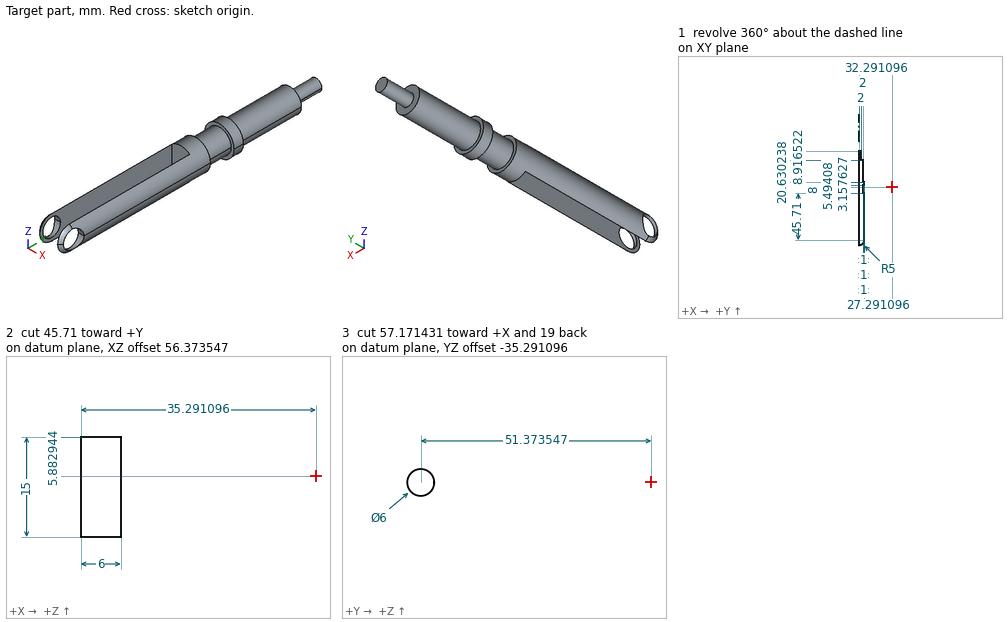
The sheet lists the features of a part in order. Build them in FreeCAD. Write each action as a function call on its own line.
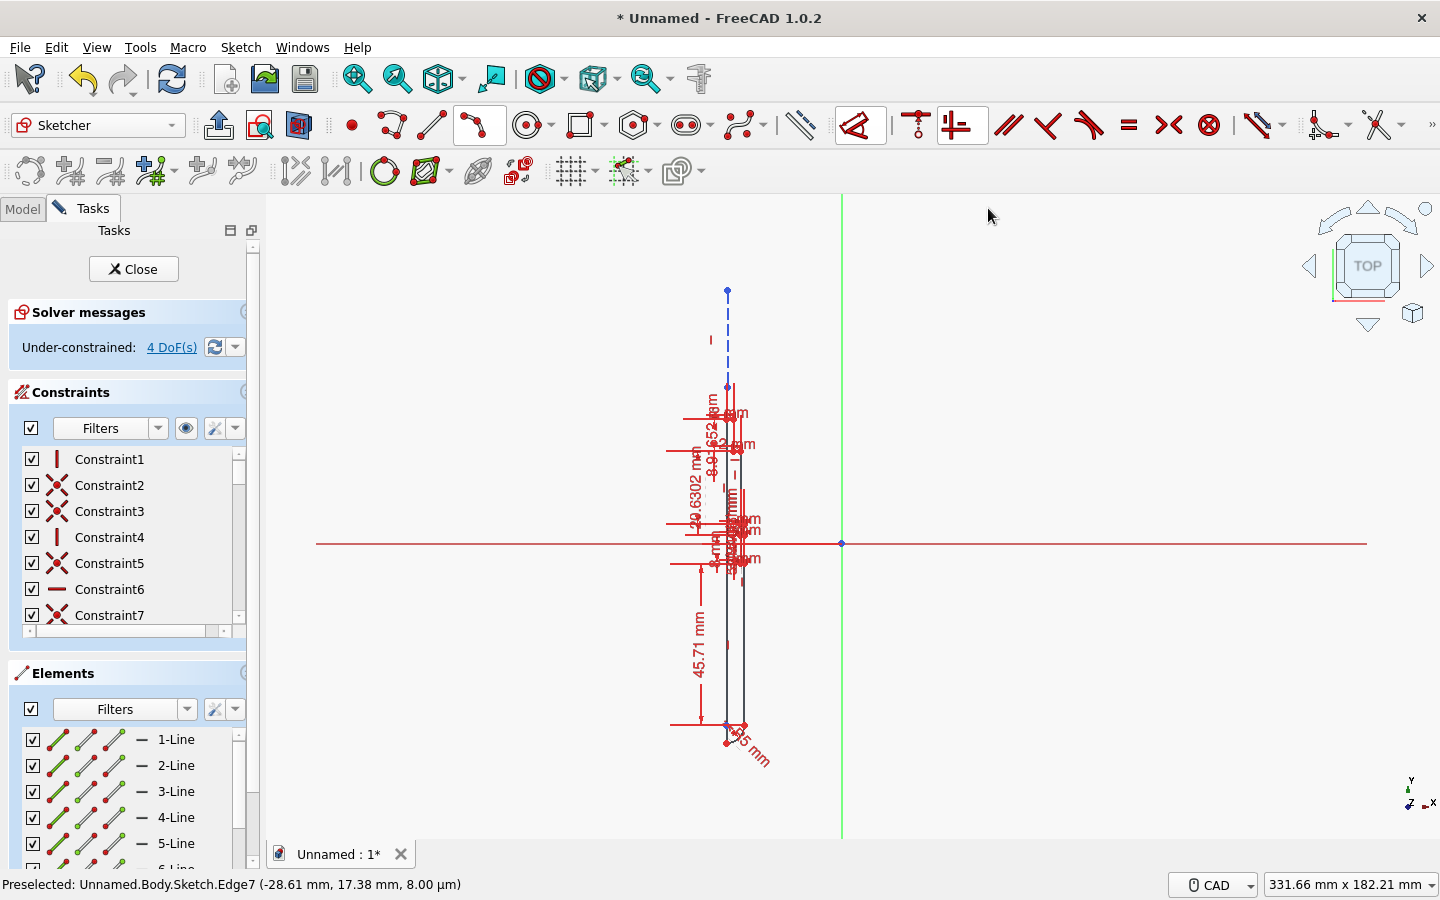
click(744, 725)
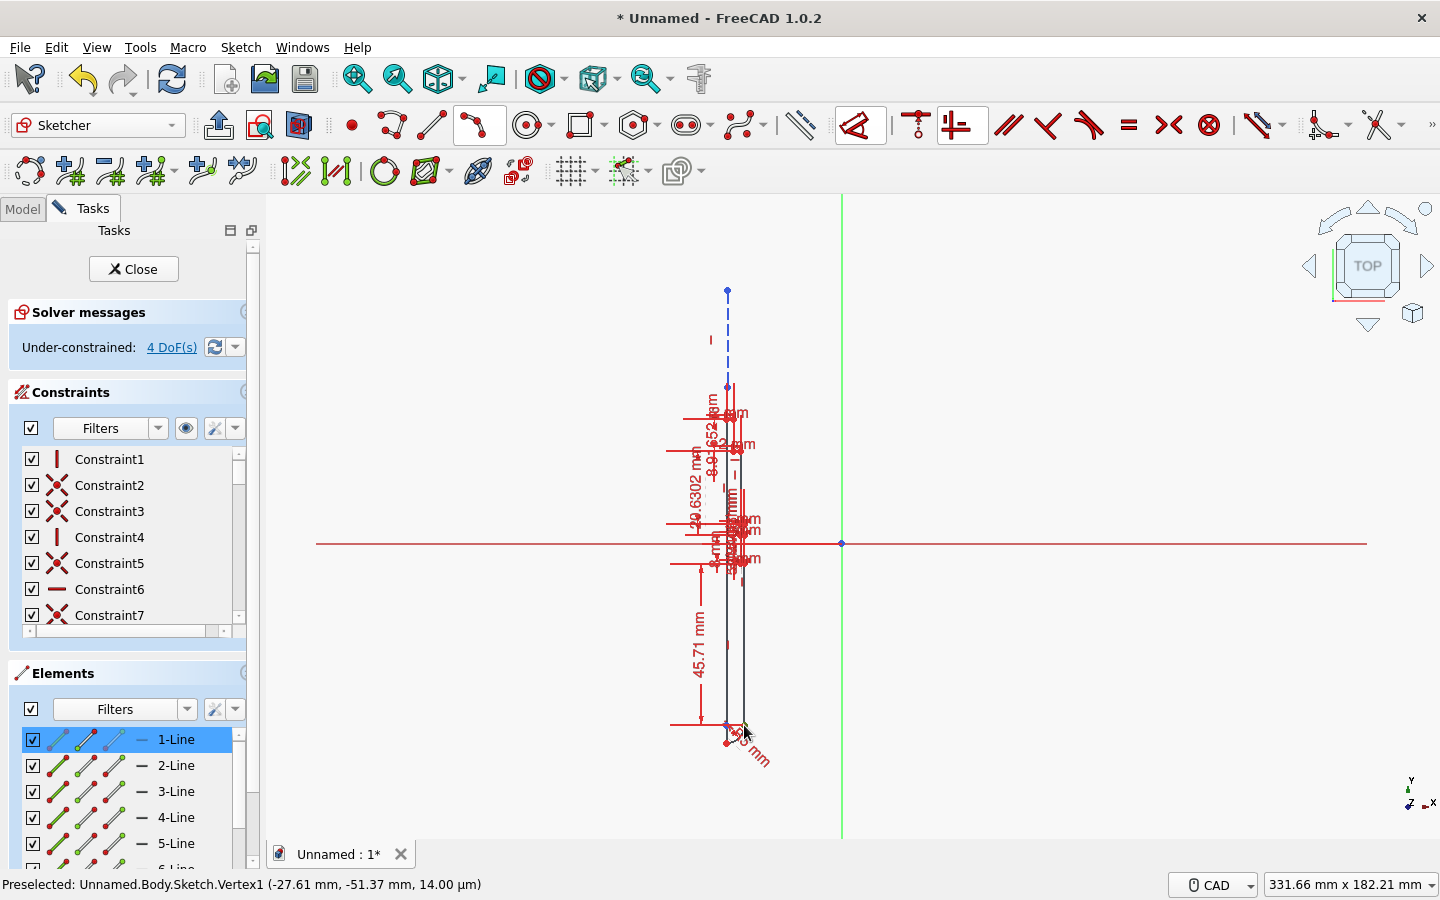
click(880, 126)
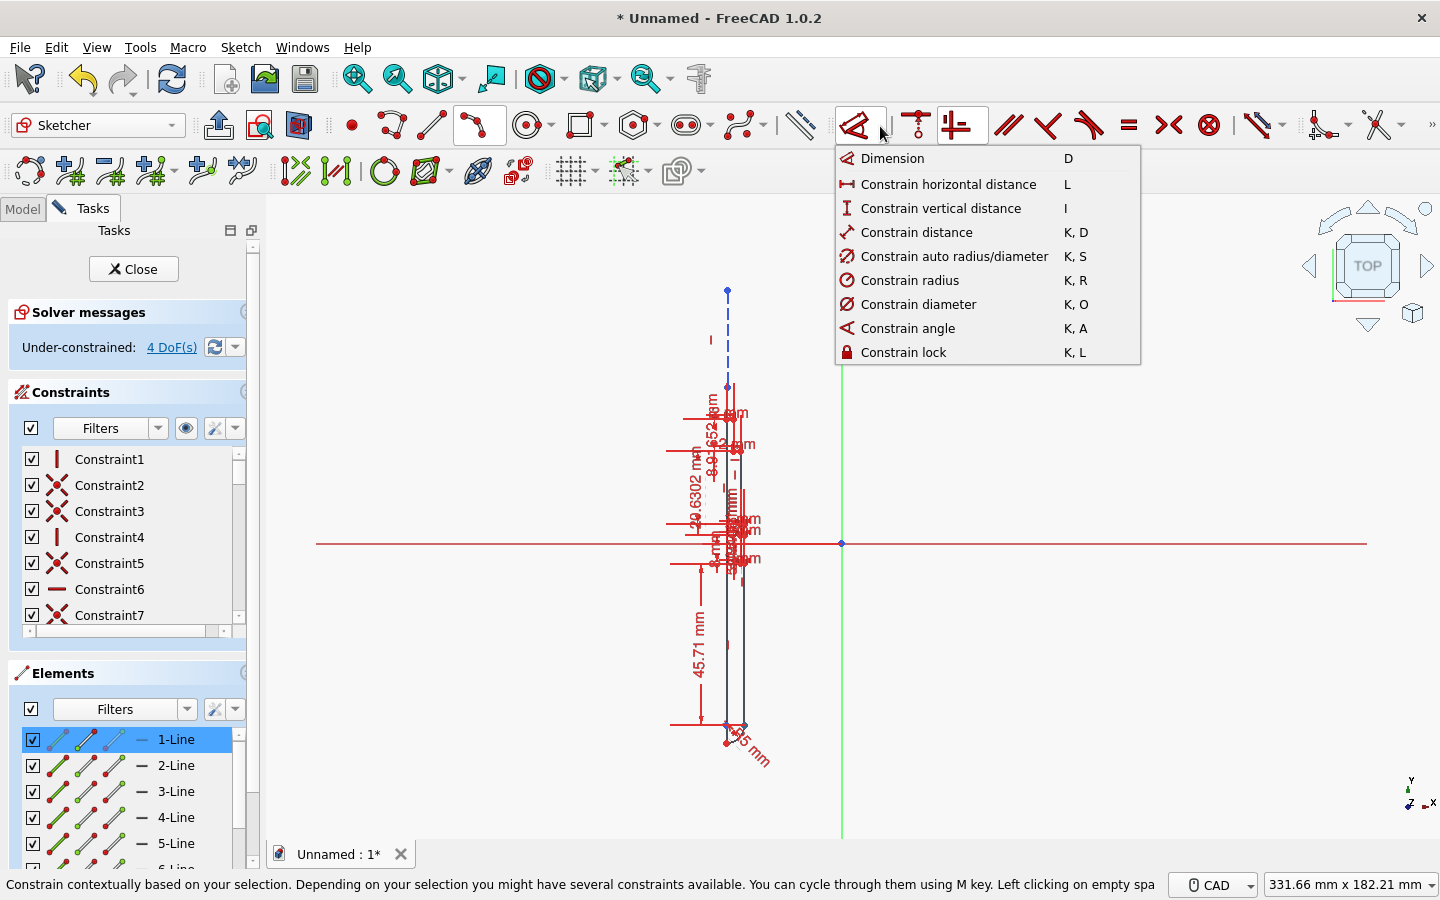
click(988, 184)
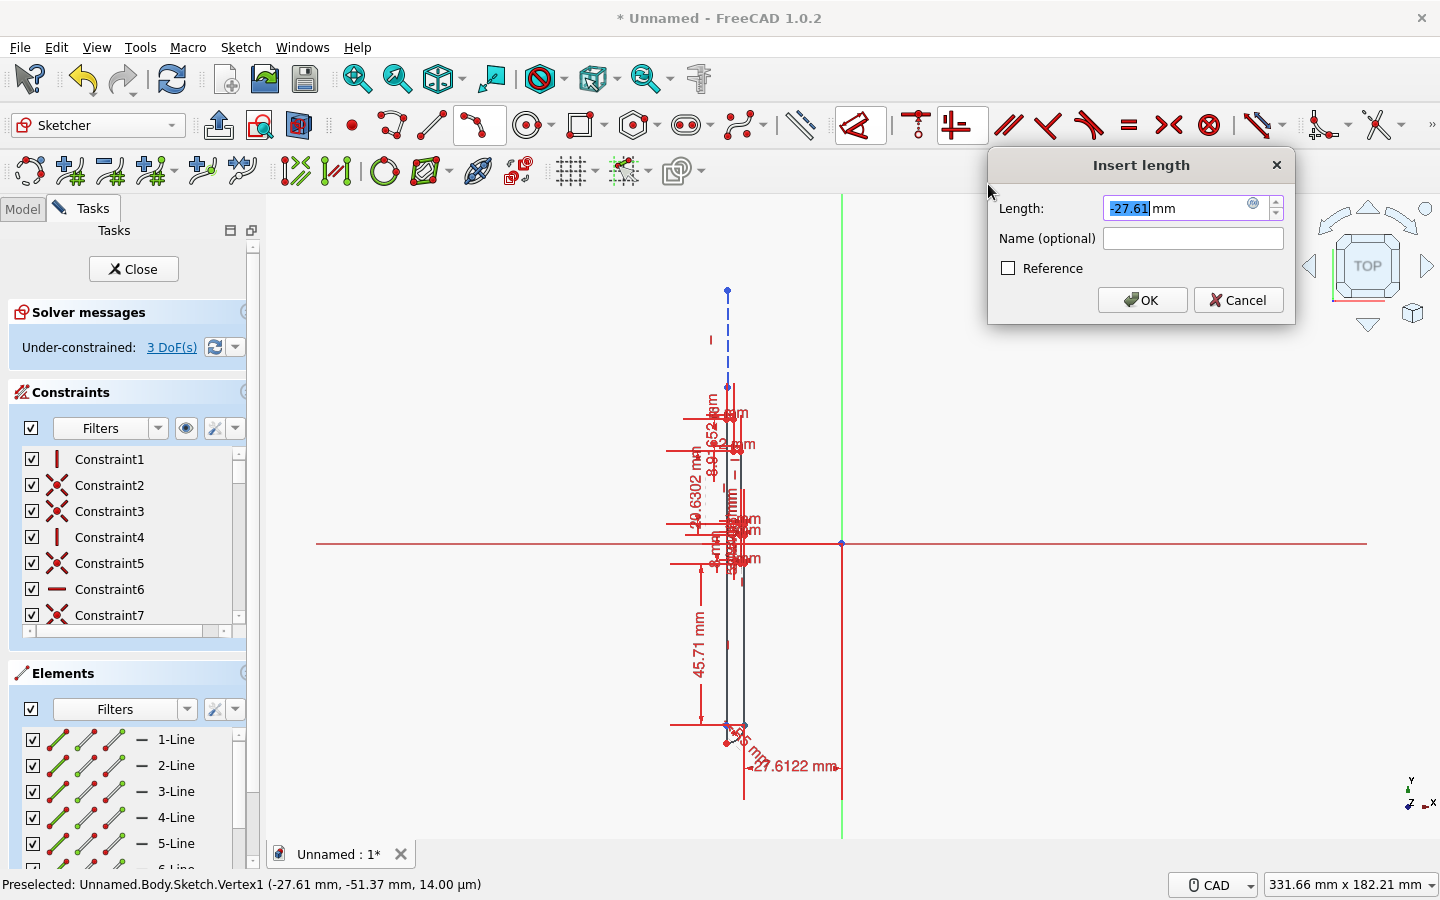
text(-27.291096)
key(Return)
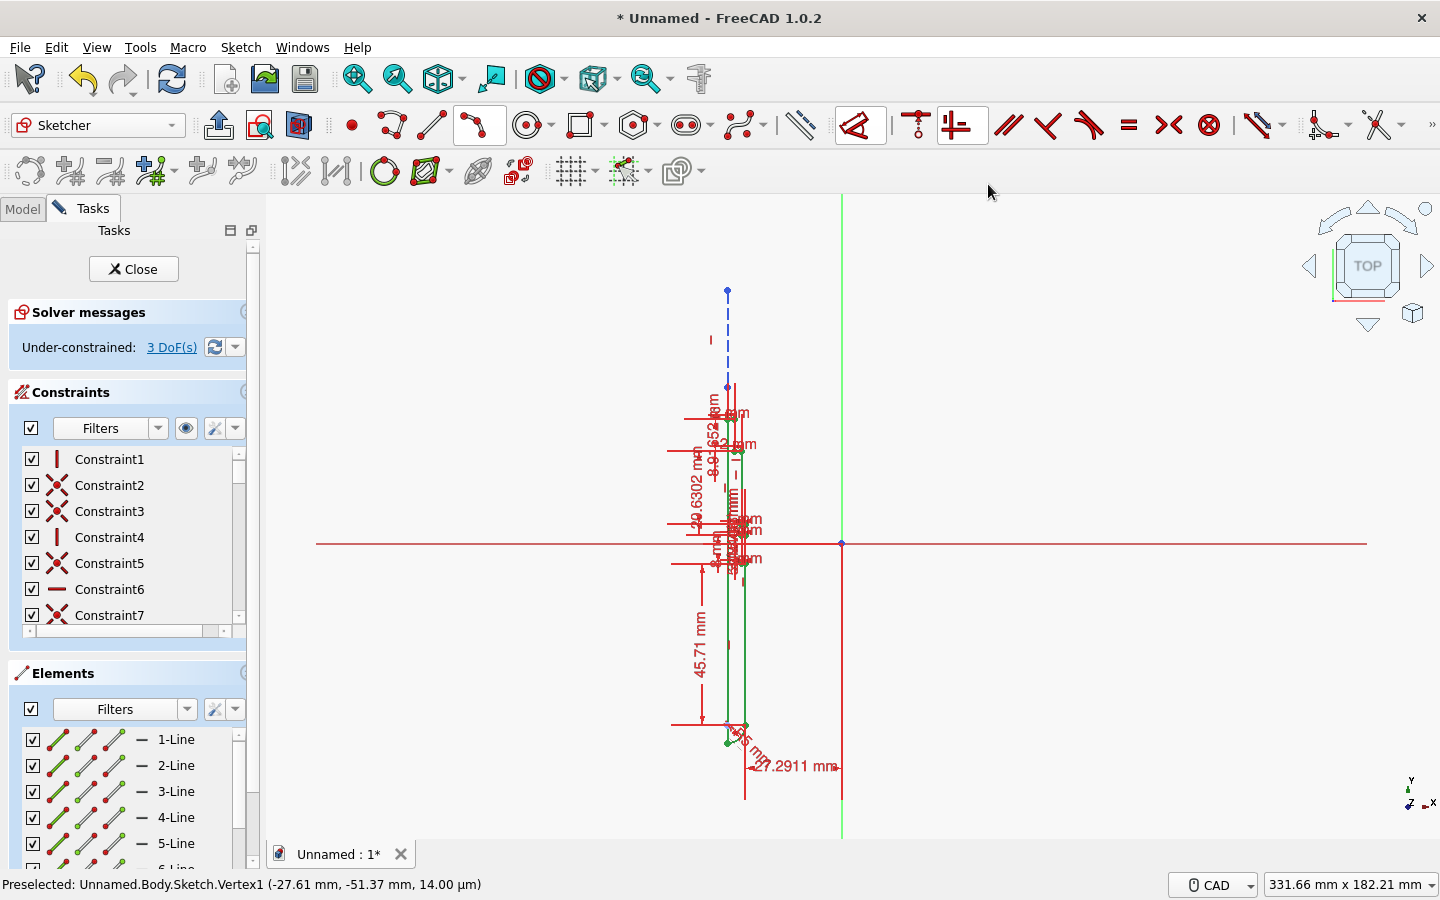
click(728, 388)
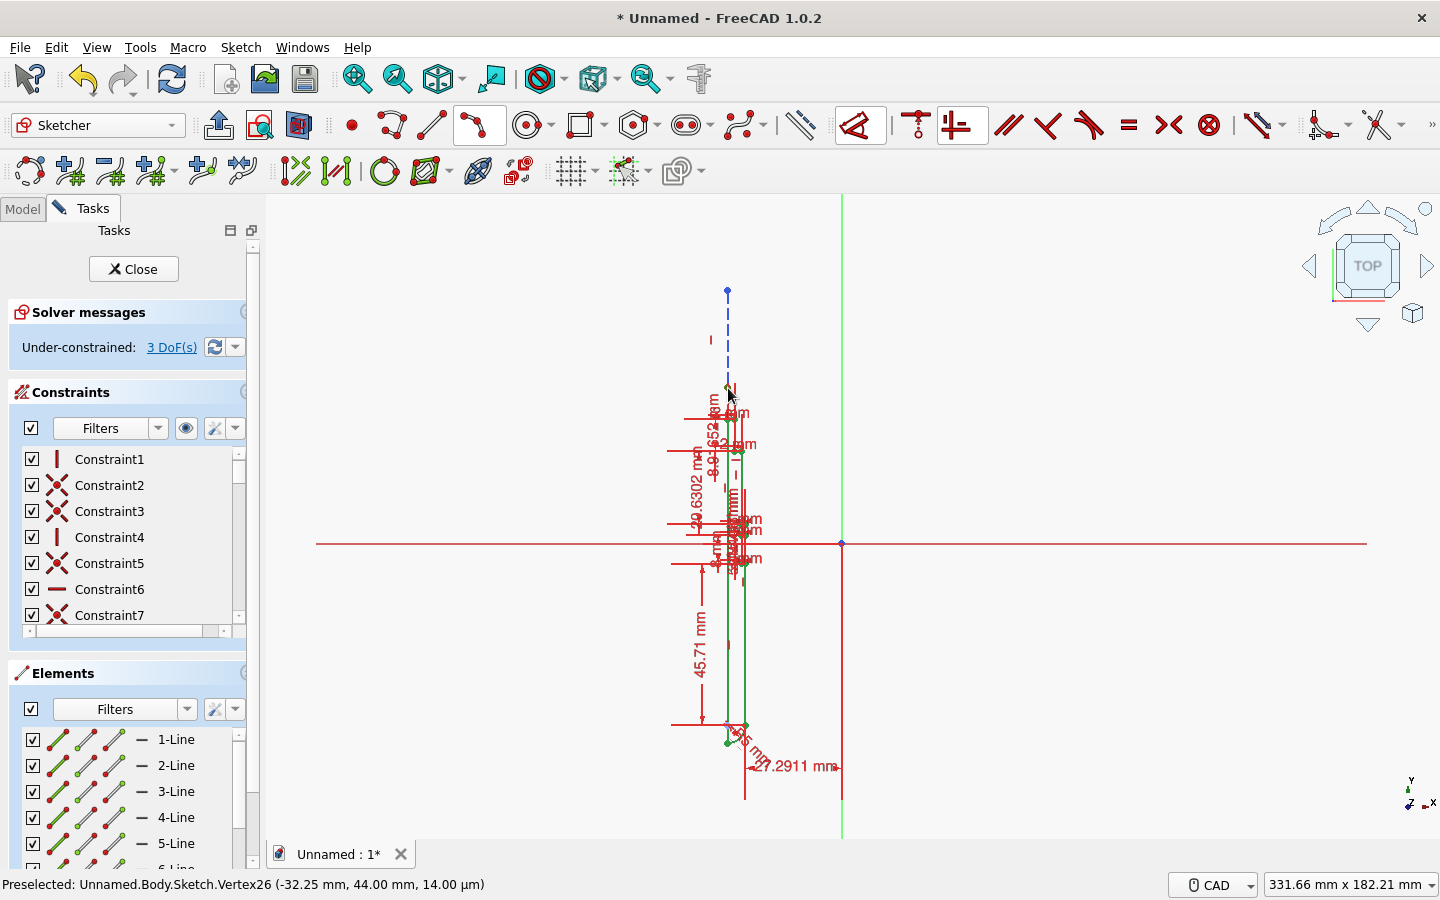
click(880, 126)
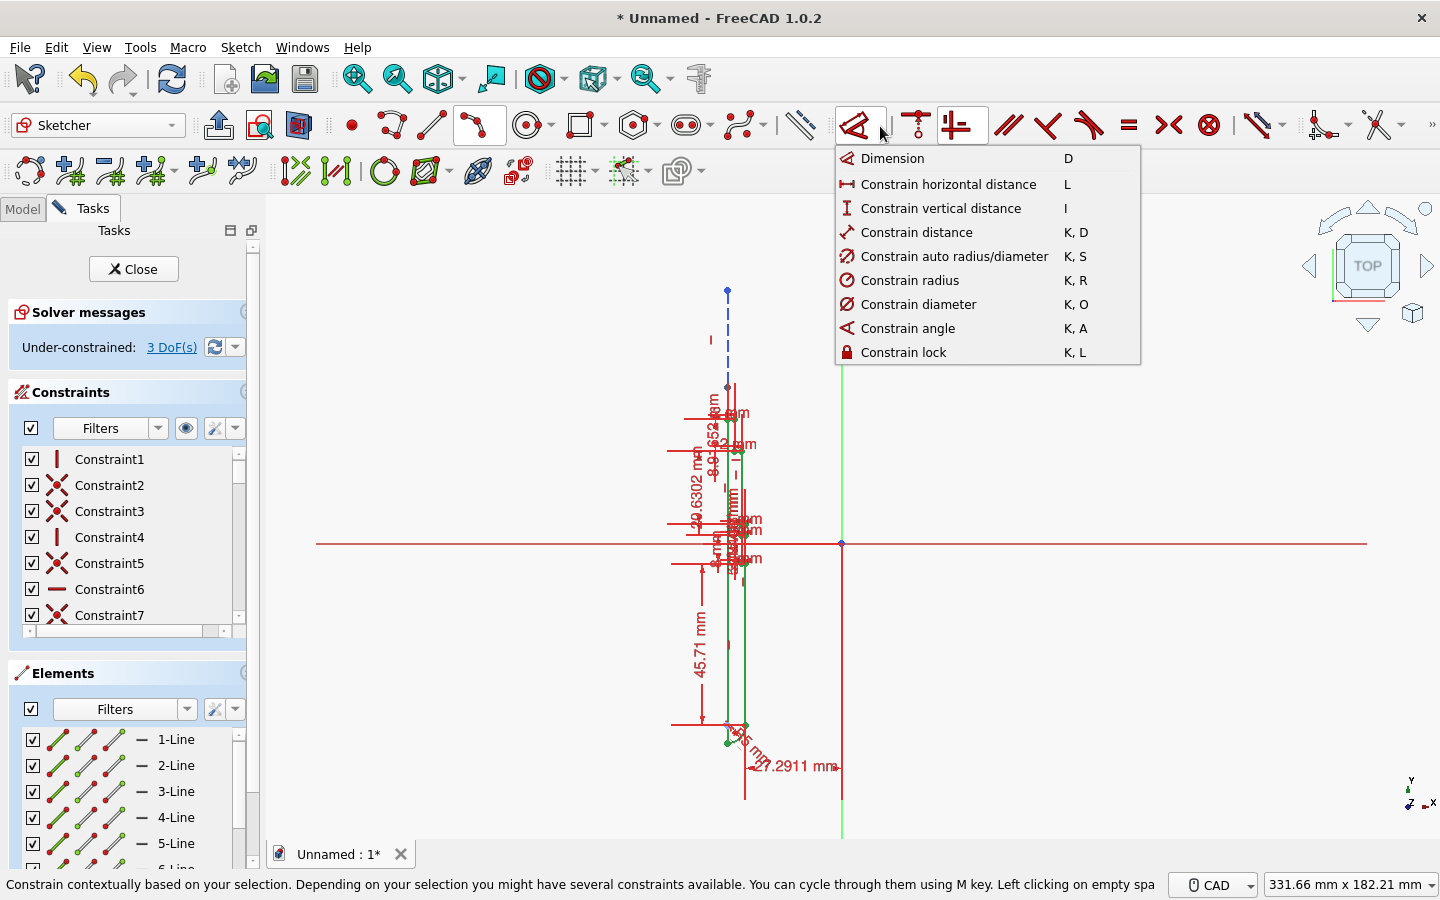
click(988, 184)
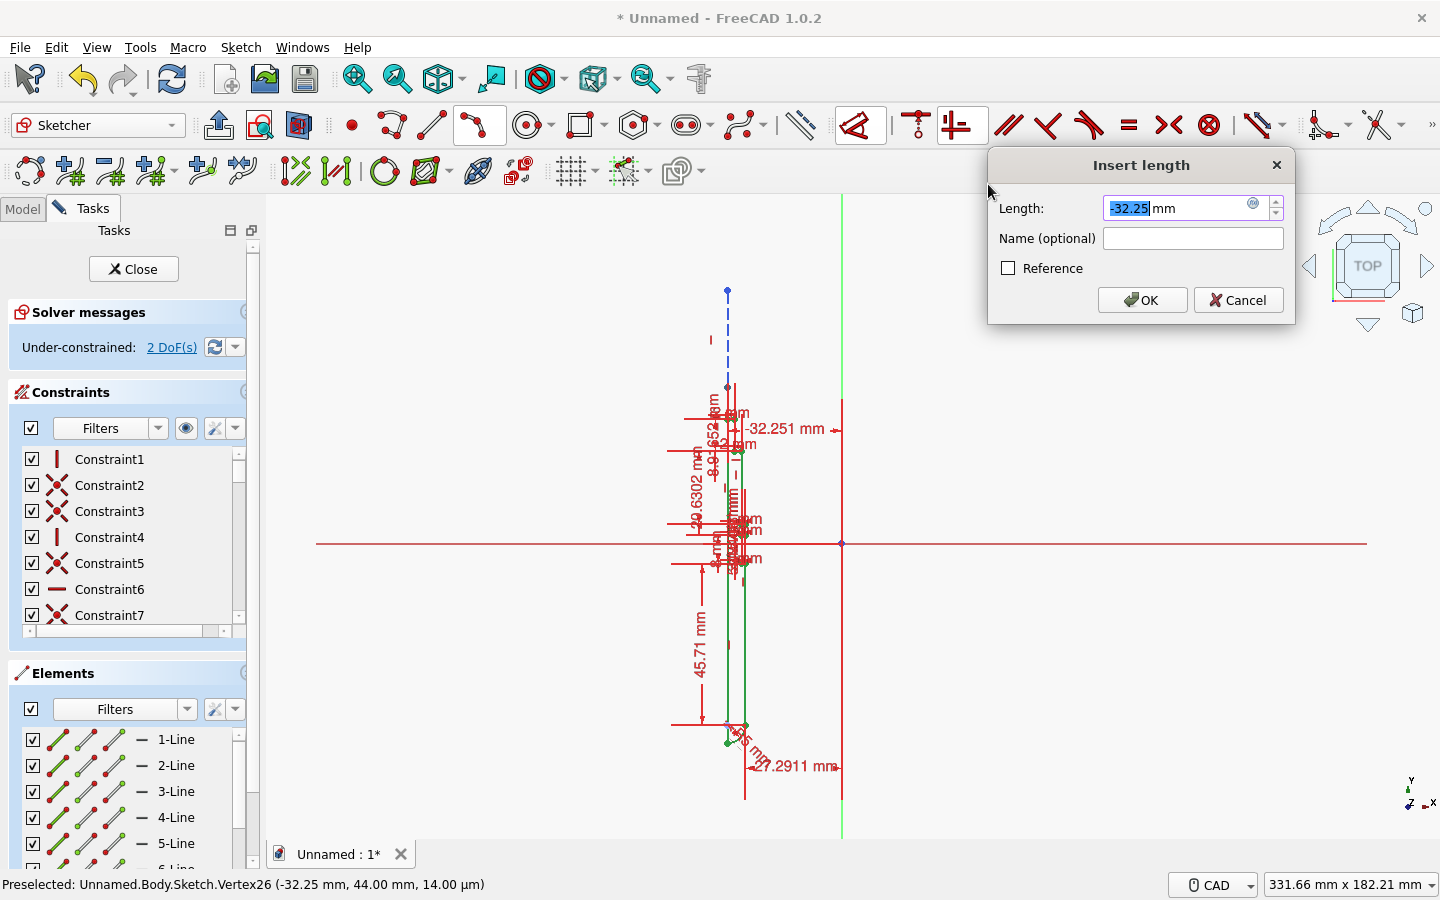
text(-32.291096)
key(Return)